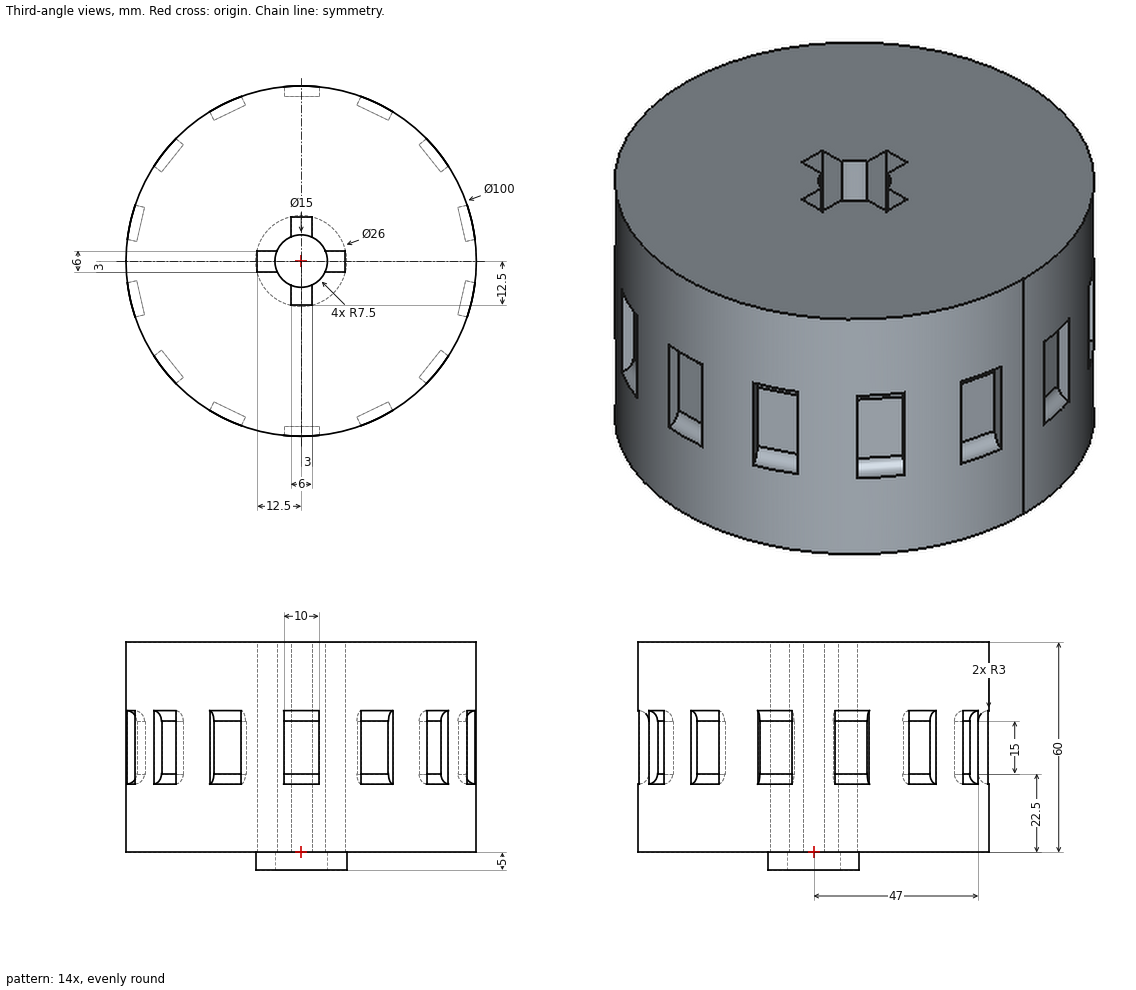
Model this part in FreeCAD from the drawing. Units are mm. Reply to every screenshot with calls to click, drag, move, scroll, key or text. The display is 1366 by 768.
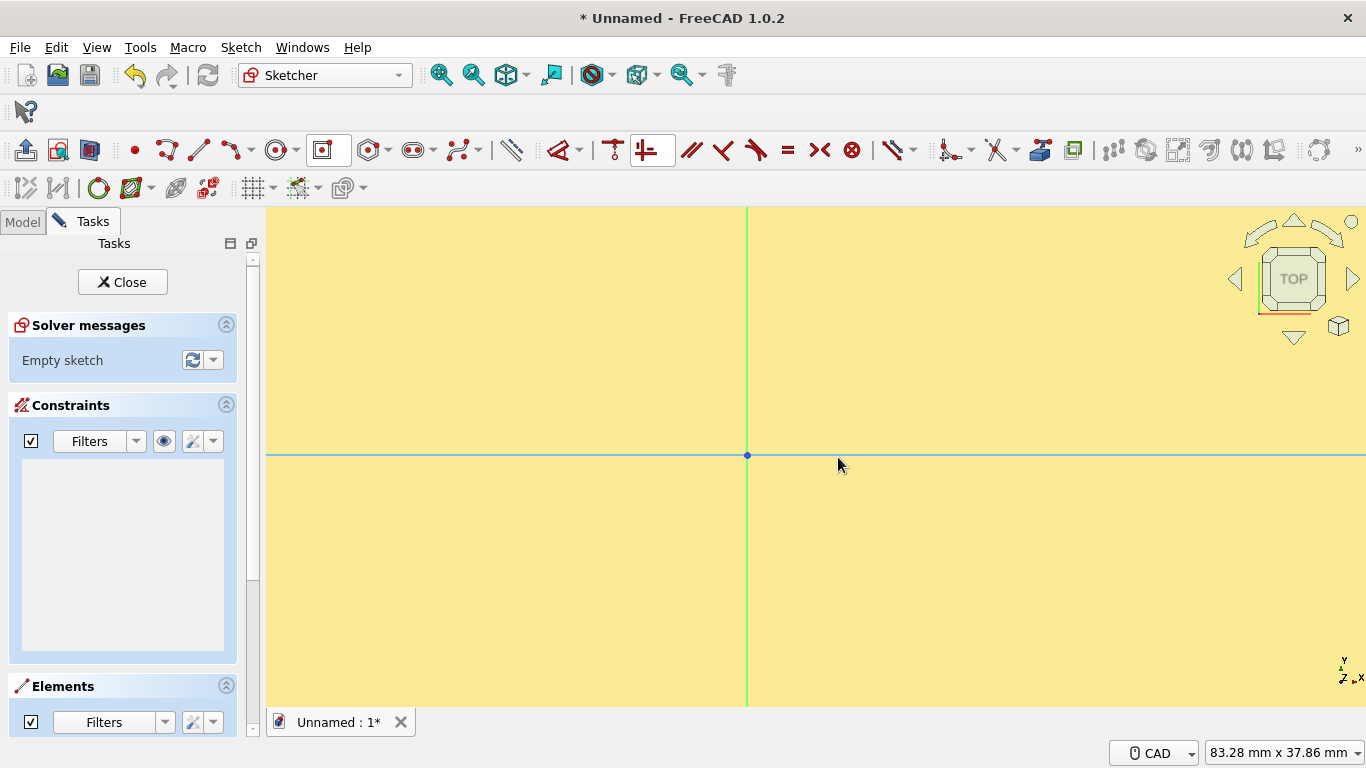
key(g)
key(c)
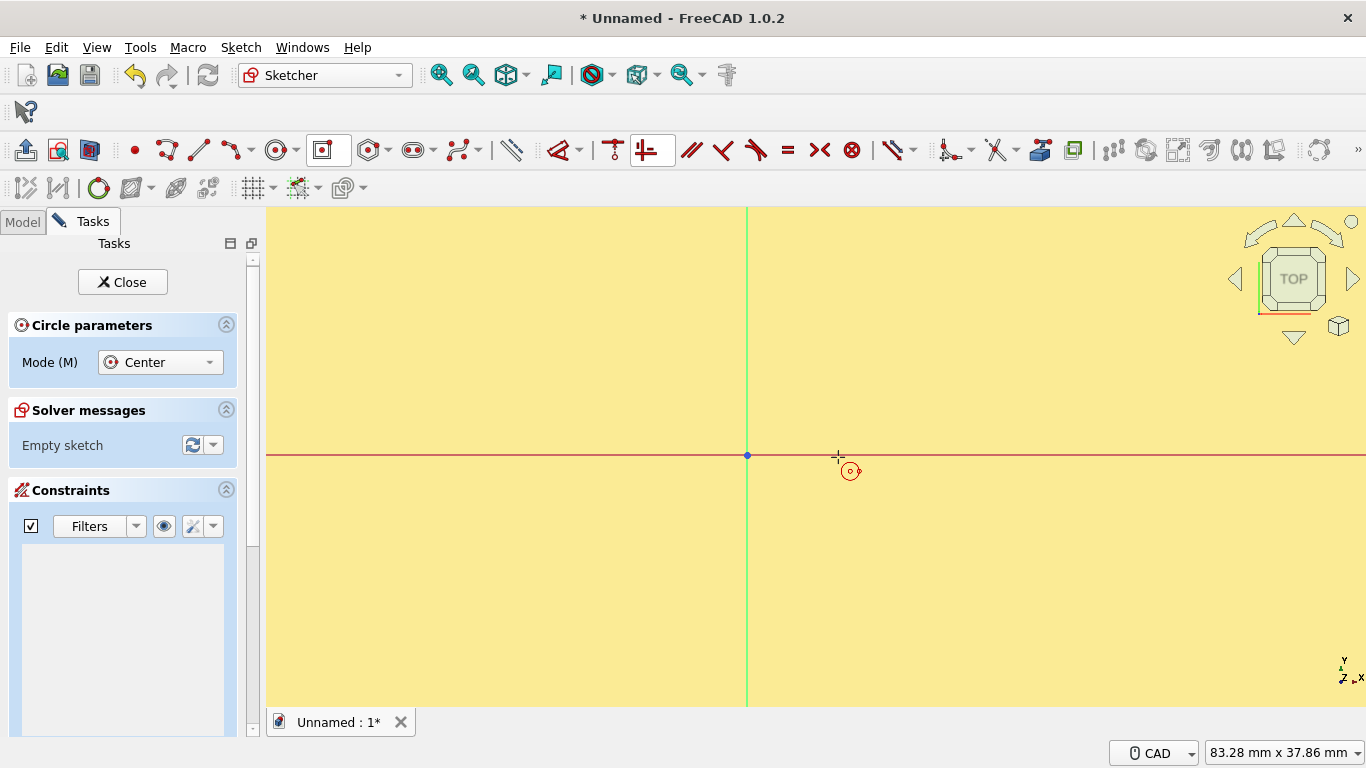
click(747, 455)
click(869, 334)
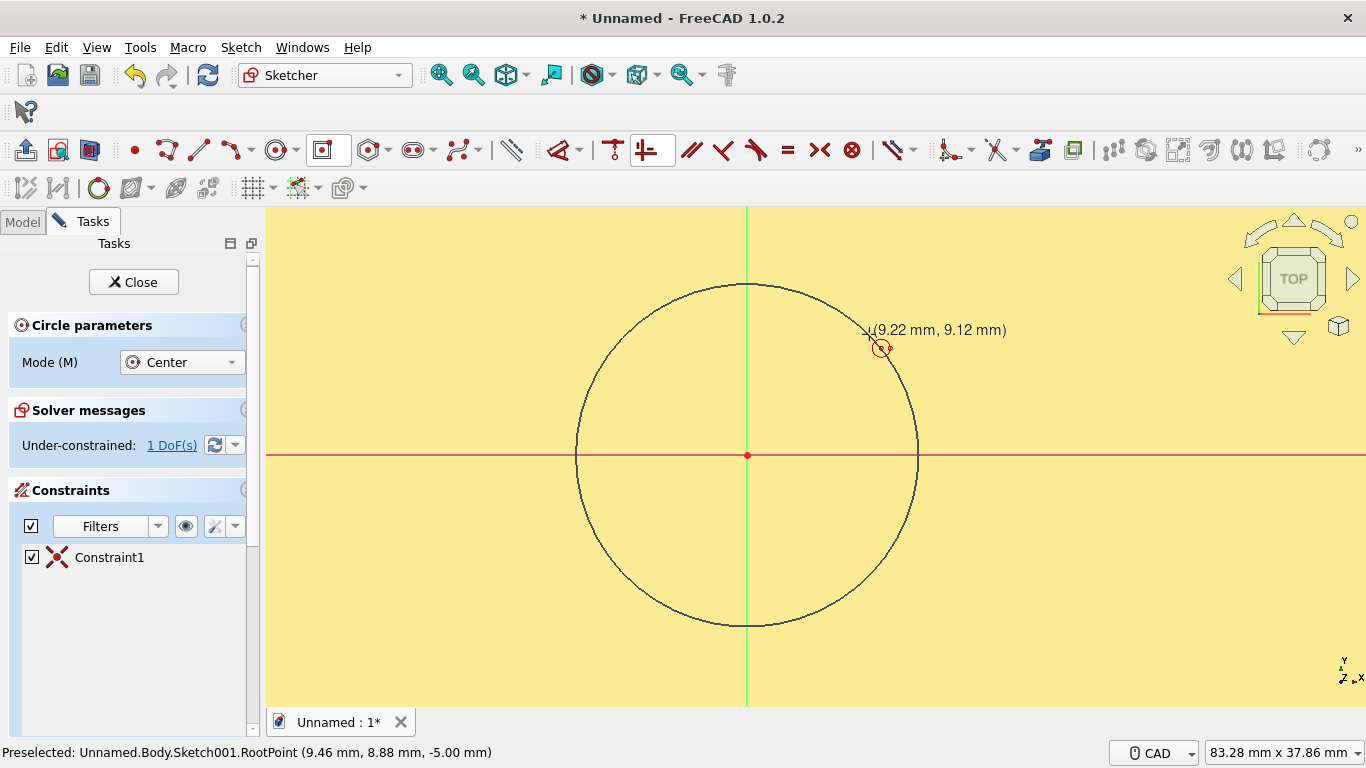
click(747, 455)
click(817, 385)
key(Escape)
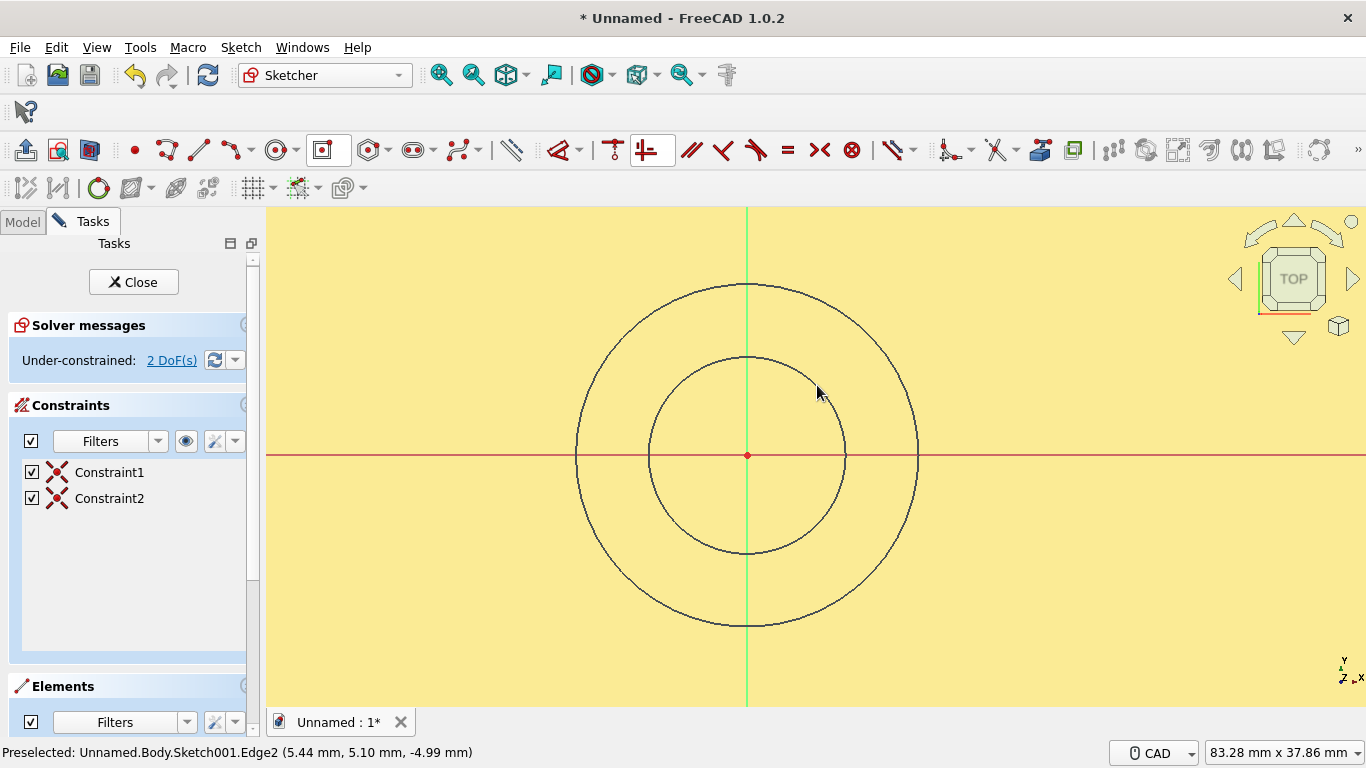
click(558, 150)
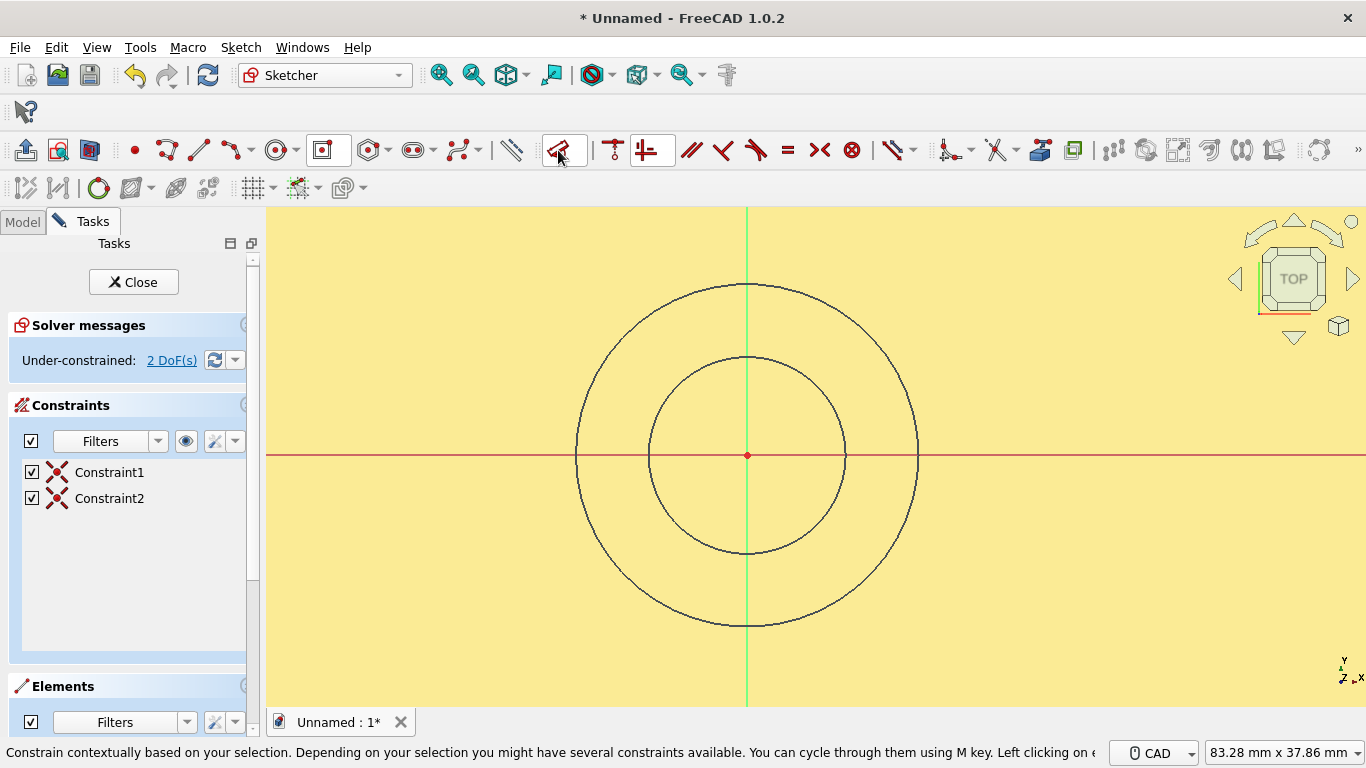
click(868, 334)
click(891, 311)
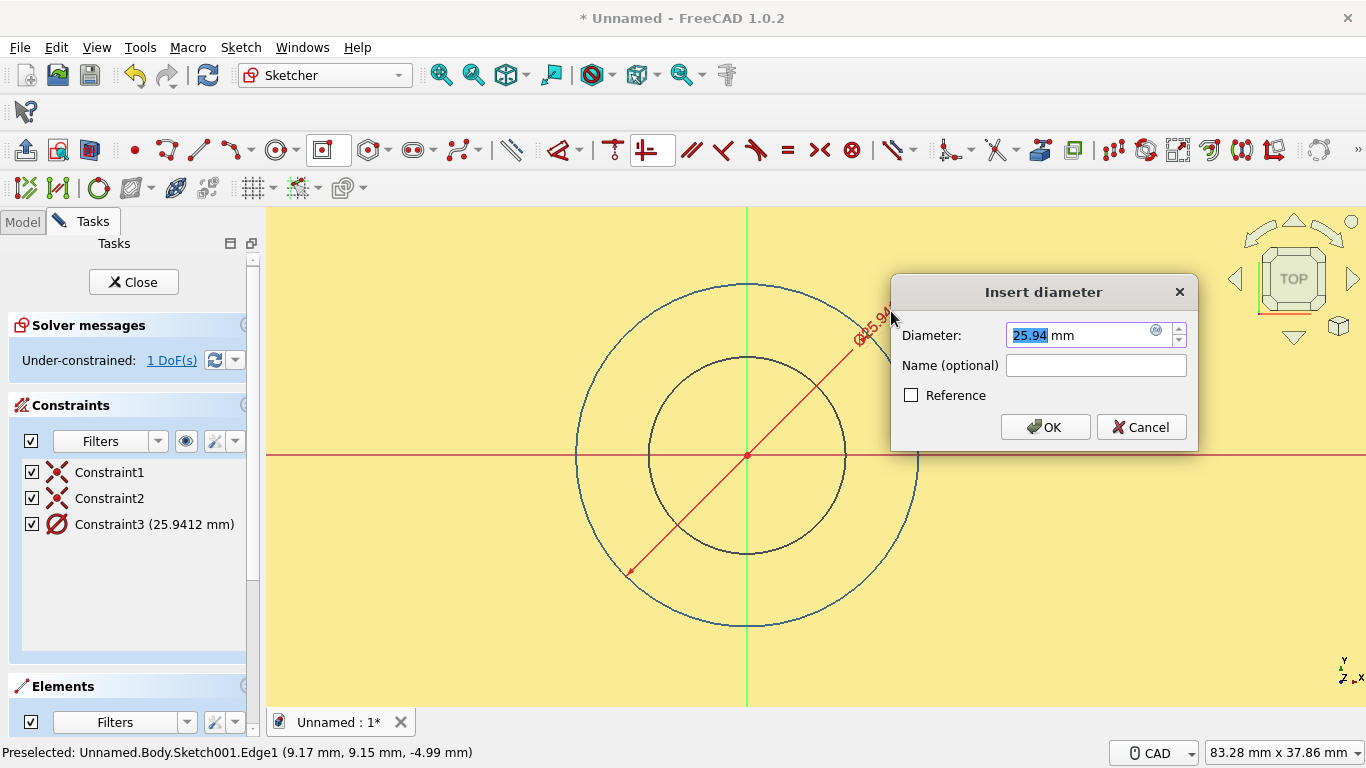
text(26)
key(Return)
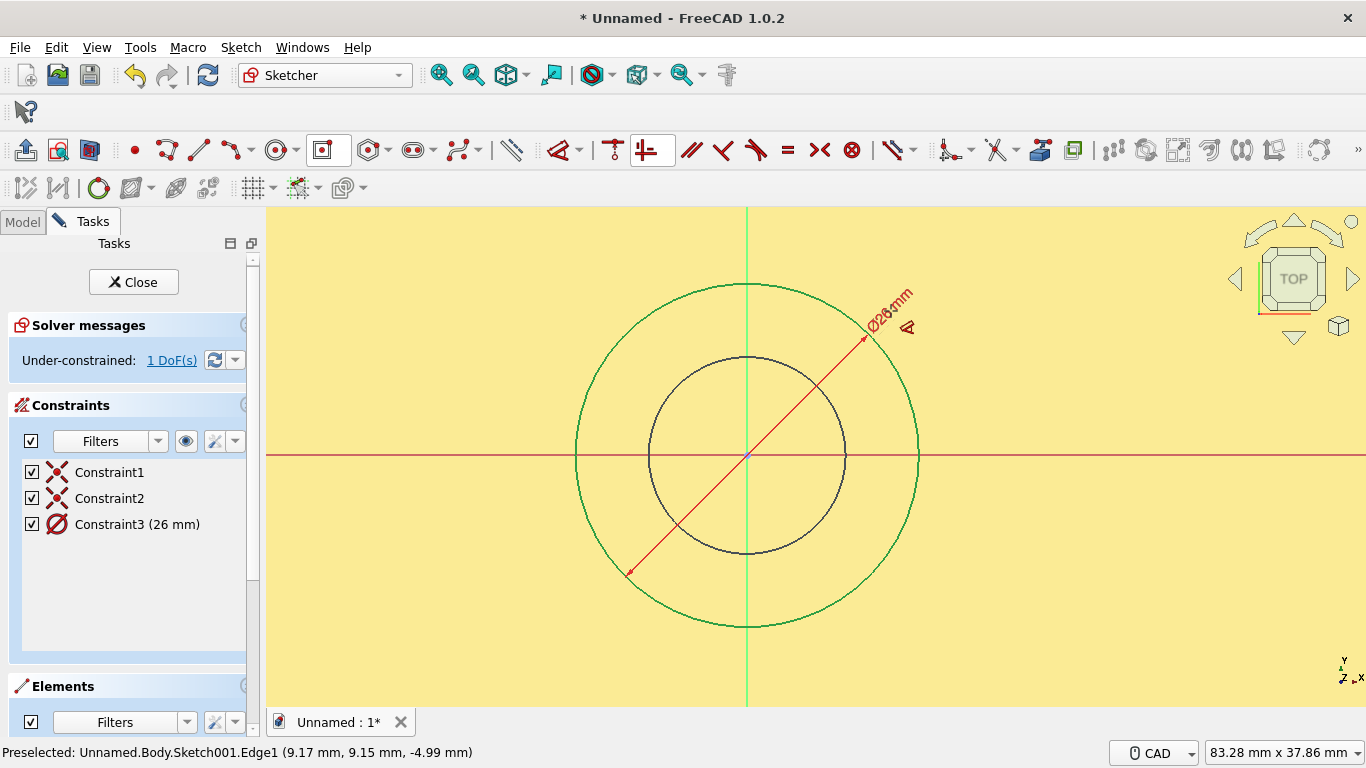
click(817, 386)
click(840, 363)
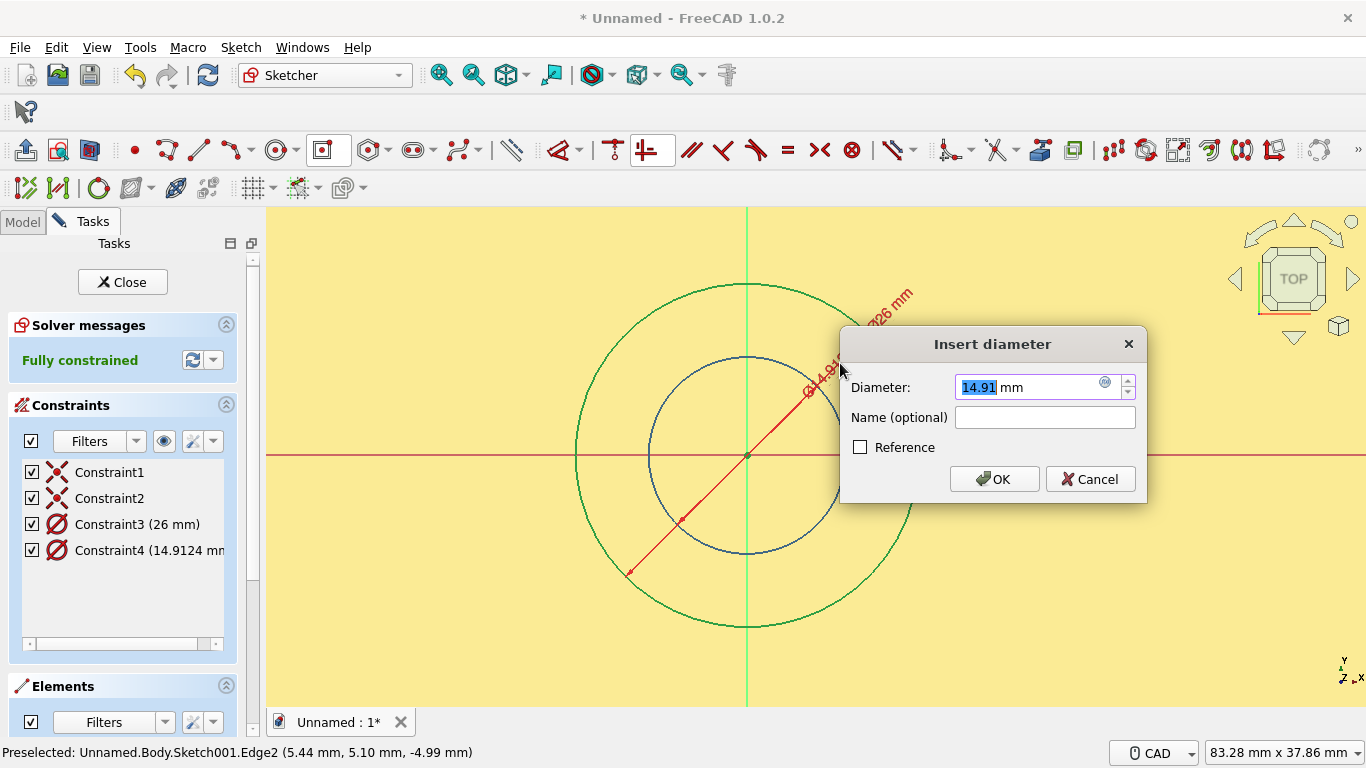
text(15)
key(Return)
key(Escape)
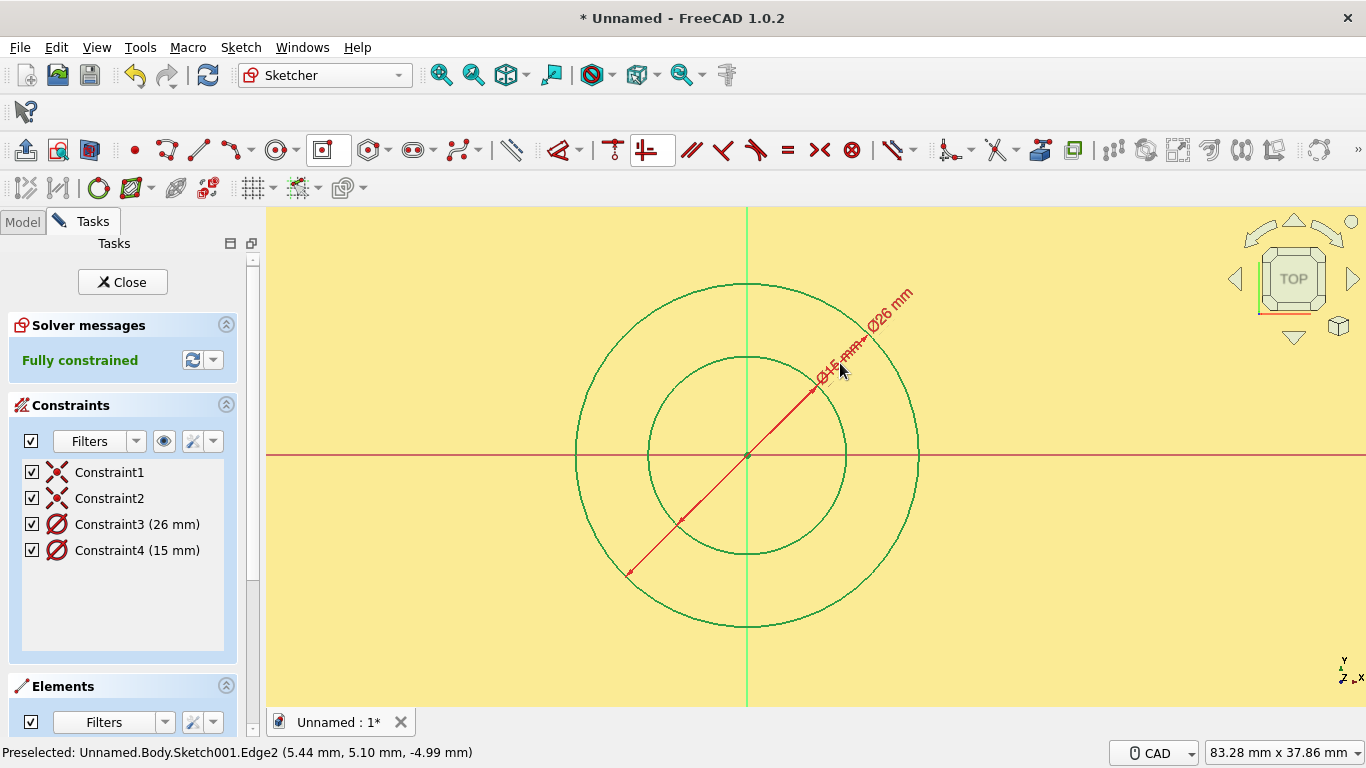
click(123, 282)